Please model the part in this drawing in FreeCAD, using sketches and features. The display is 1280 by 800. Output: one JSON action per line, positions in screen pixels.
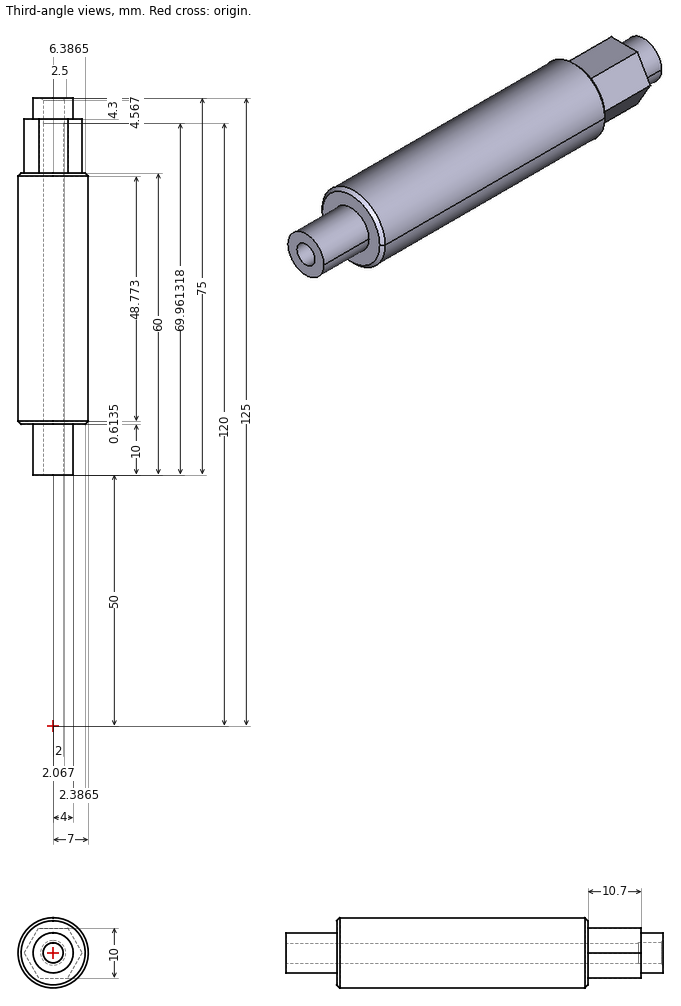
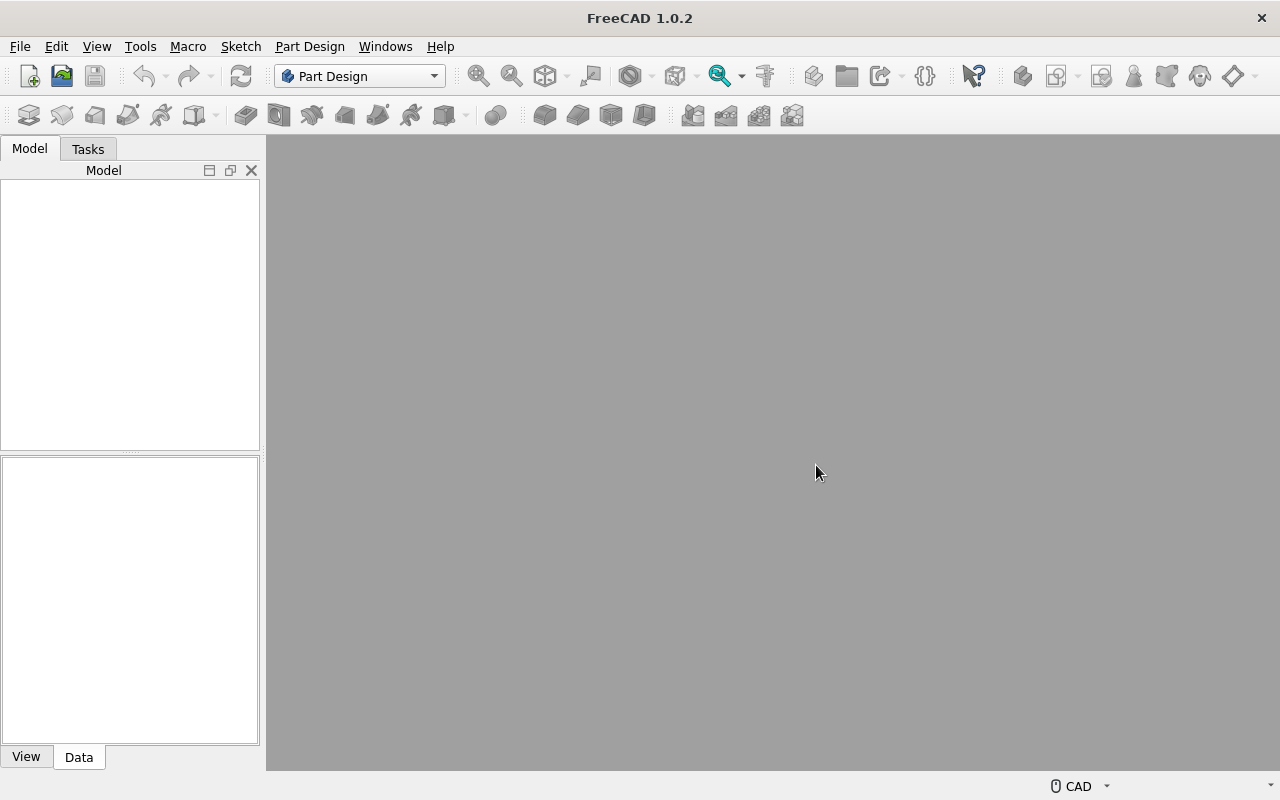
{"action": "left_click", "coordinate": [29, 76]}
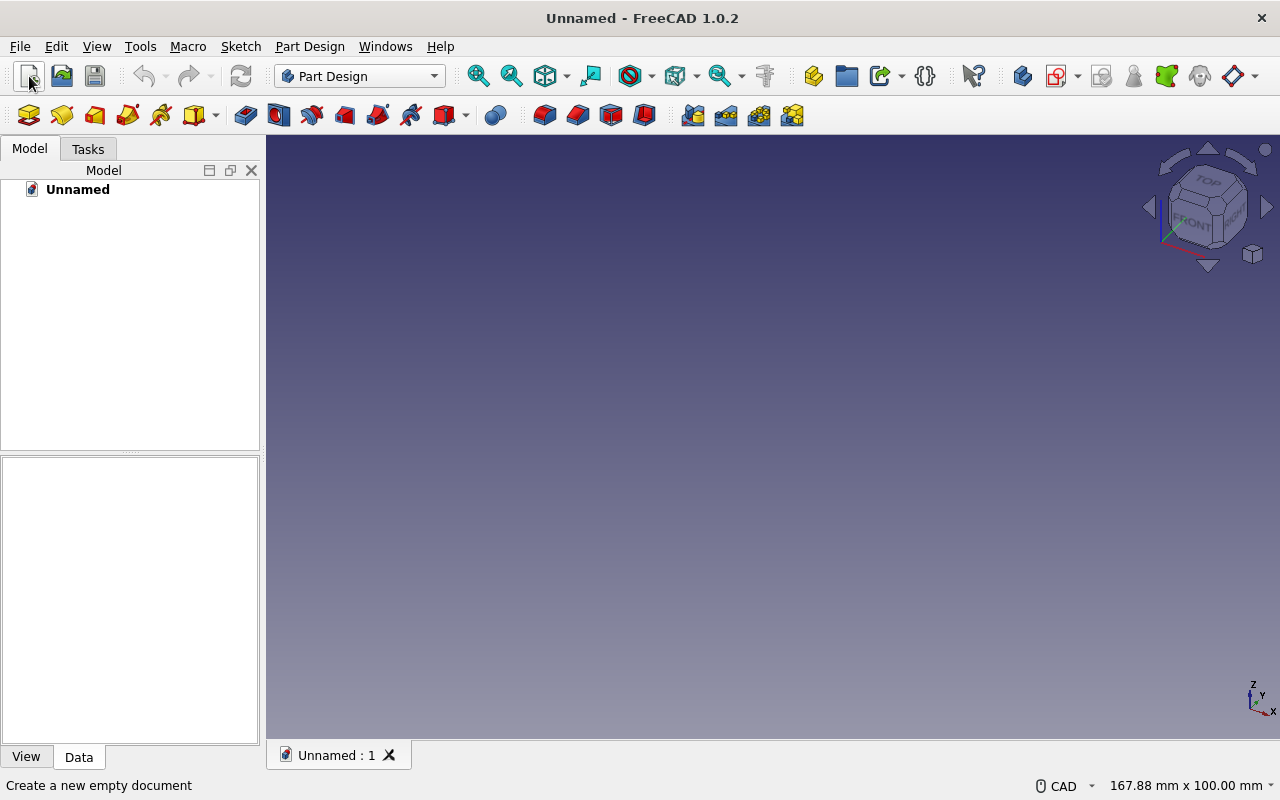
{"action": "left_click", "coordinate": [1056, 76]}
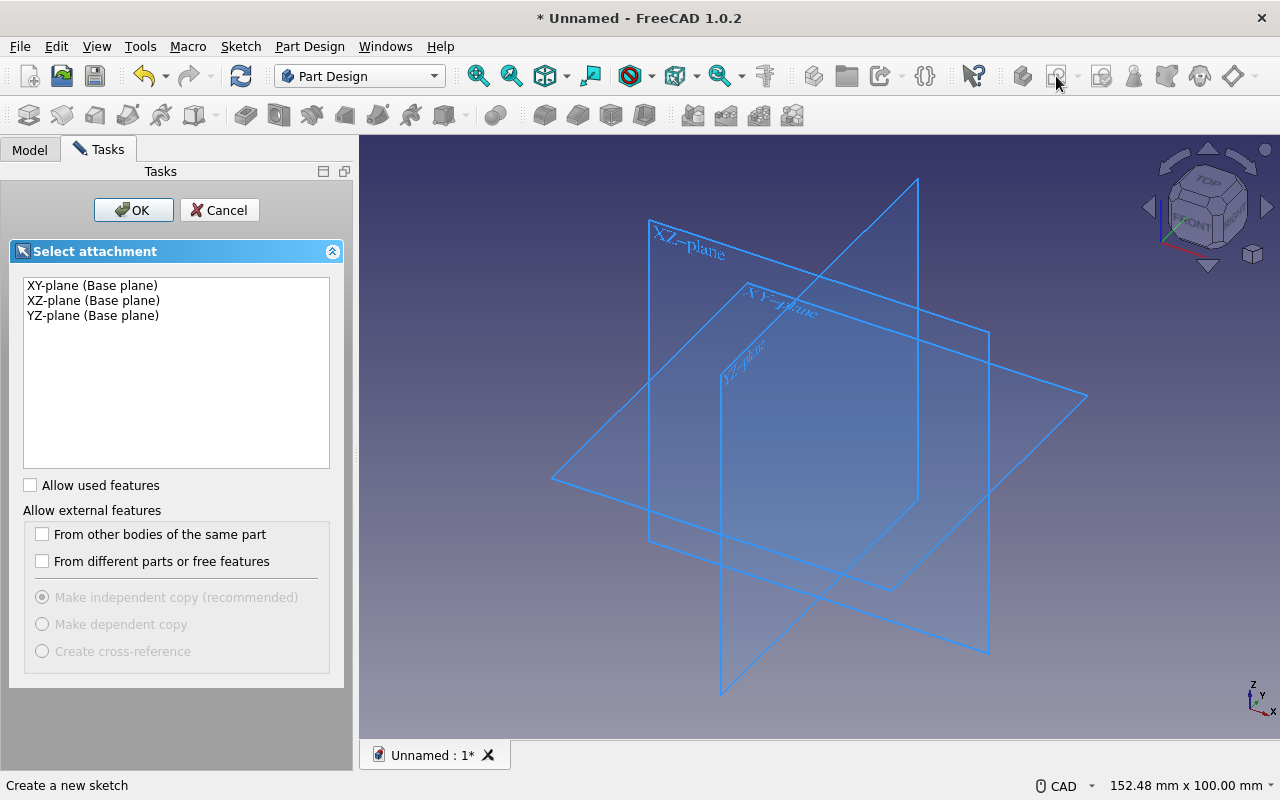
{"action": "left_click", "coordinate": [84, 286]}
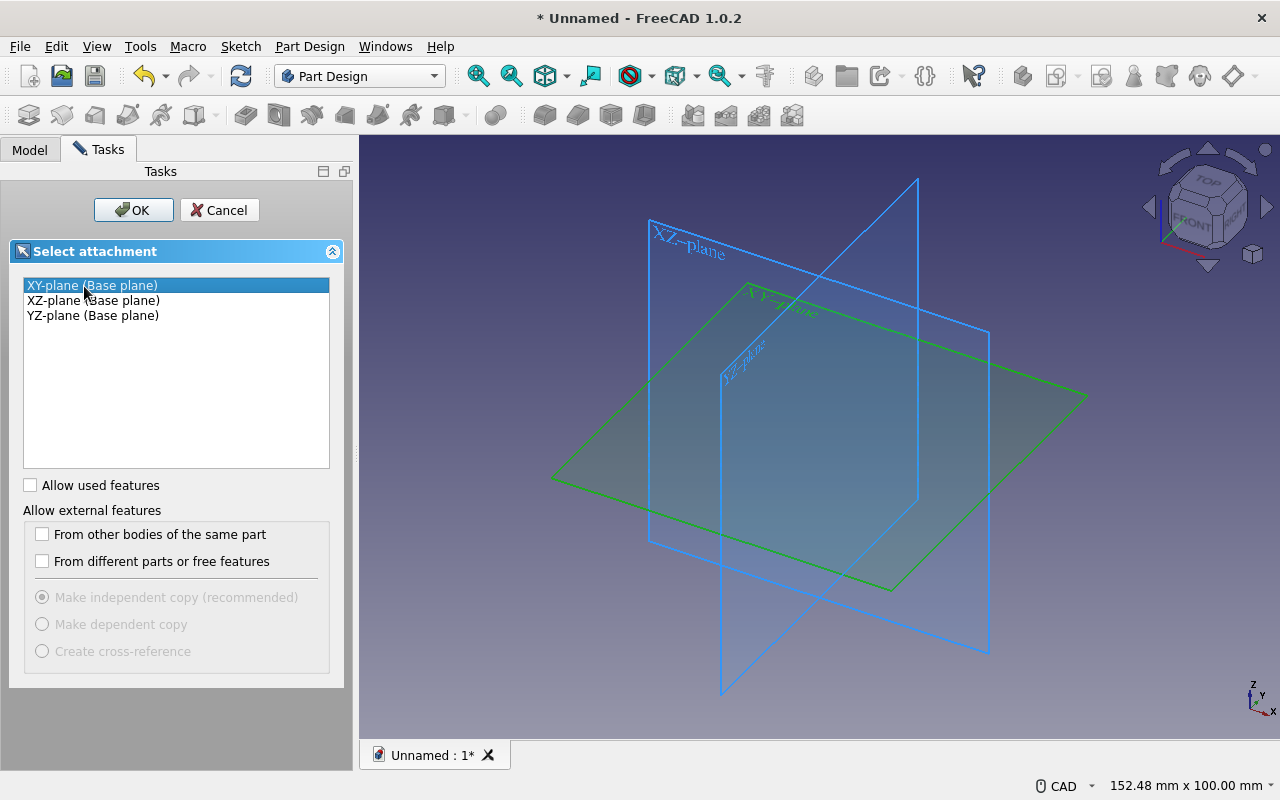
{"action": "left_click", "coordinate": [134, 210]}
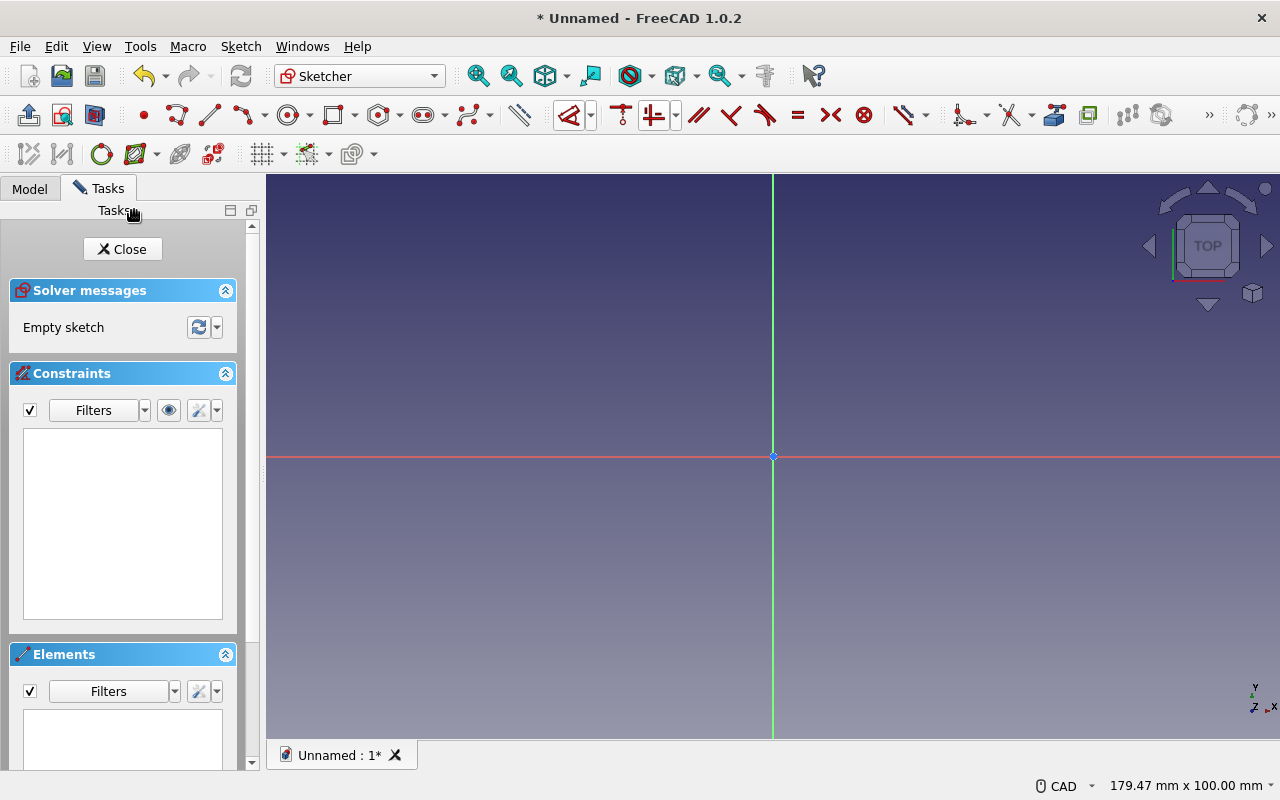
{"action": "scroll", "coordinate": [597, 711], "scroll_direction": "down", "scroll_amount": 3}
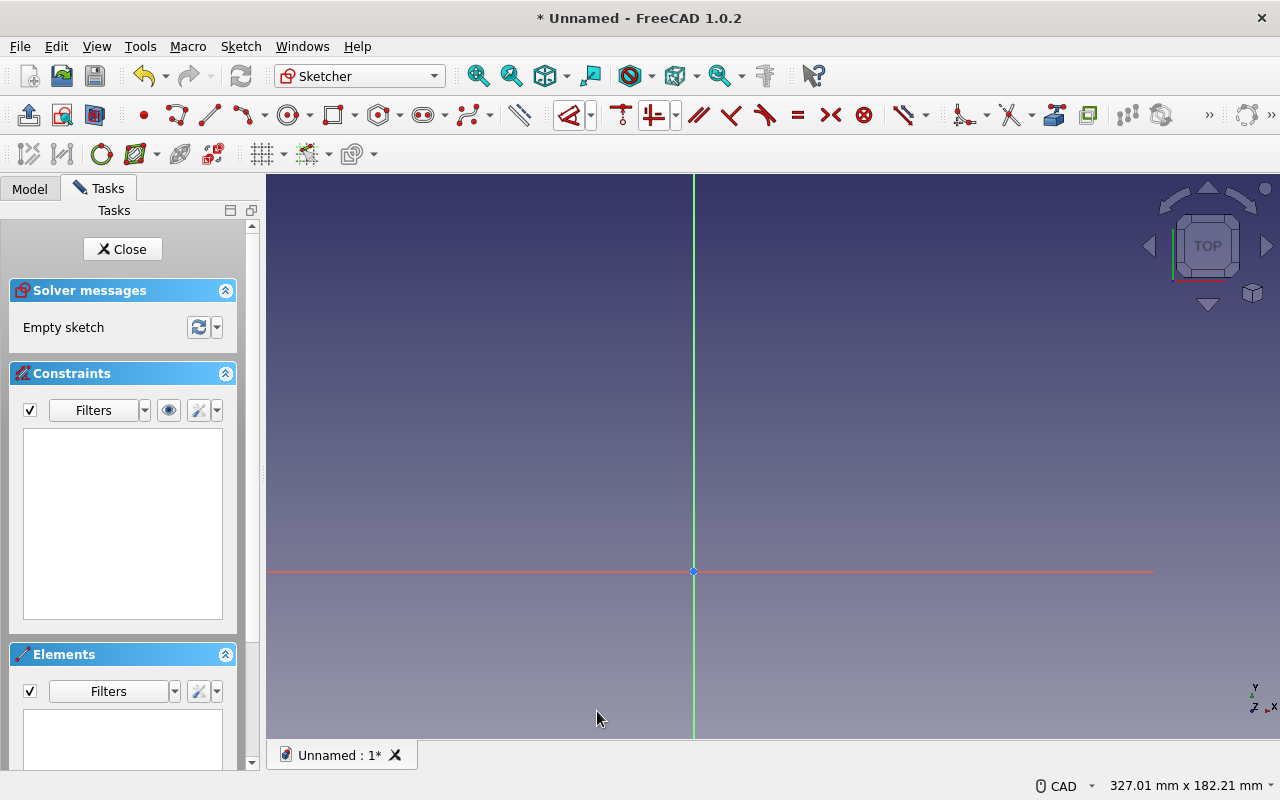
{"action": "left_click", "coordinate": [177, 116]}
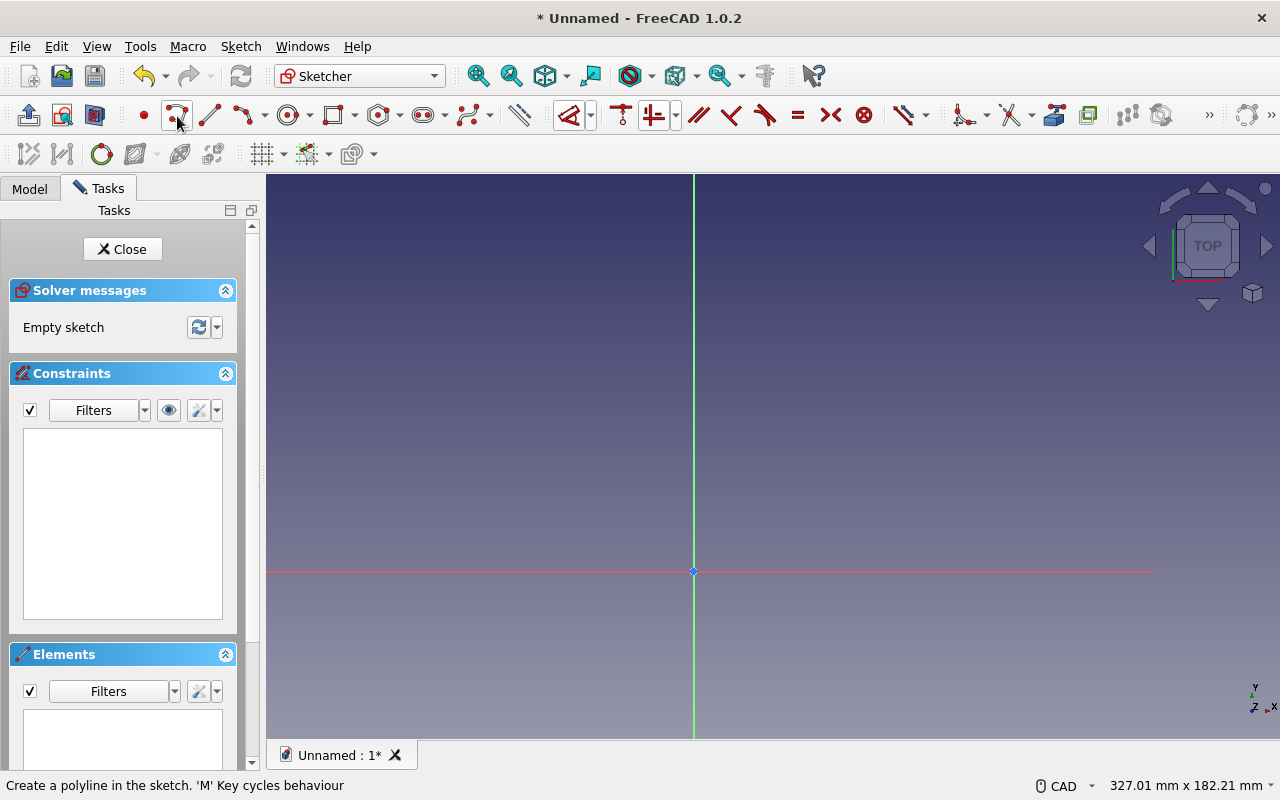
{"action": "left_click", "coordinate": [694, 417]}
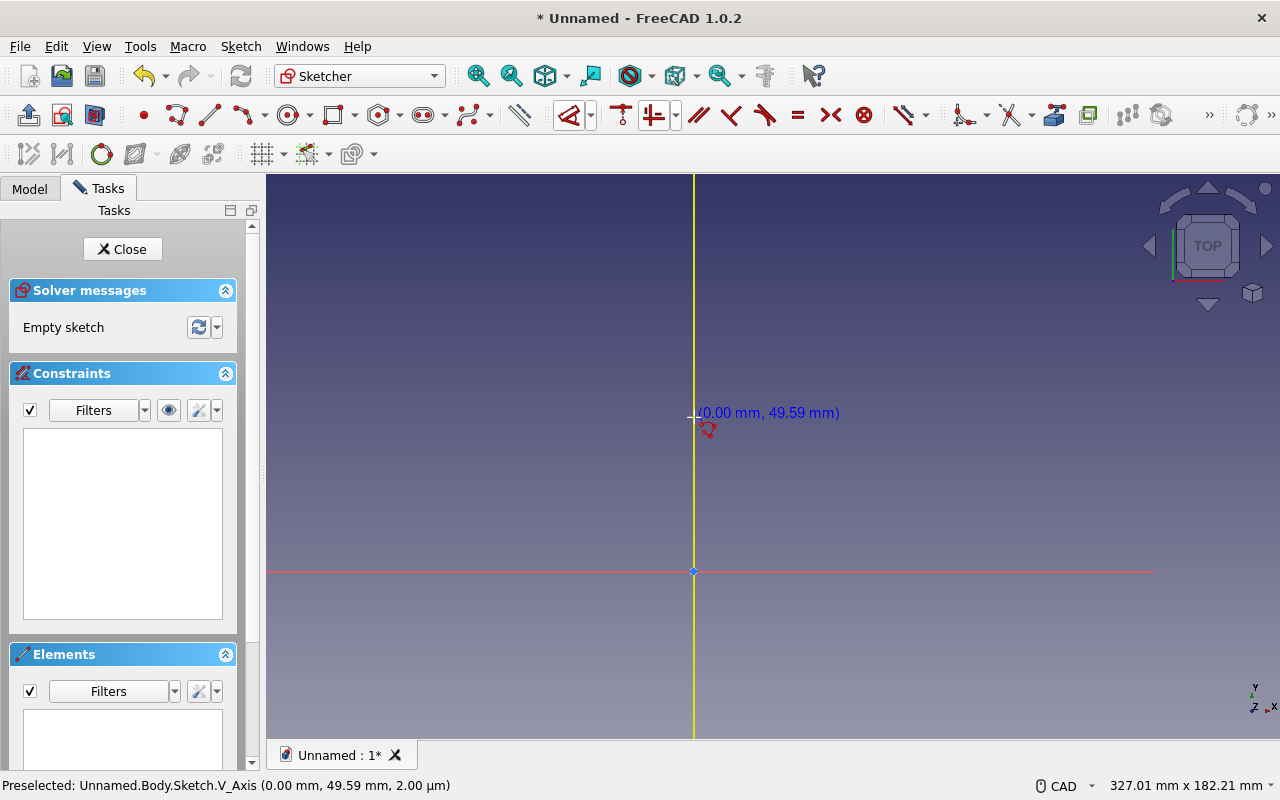
{"action": "scroll", "coordinate": [706, 417], "scroll_direction": "up", "scroll_amount": 2}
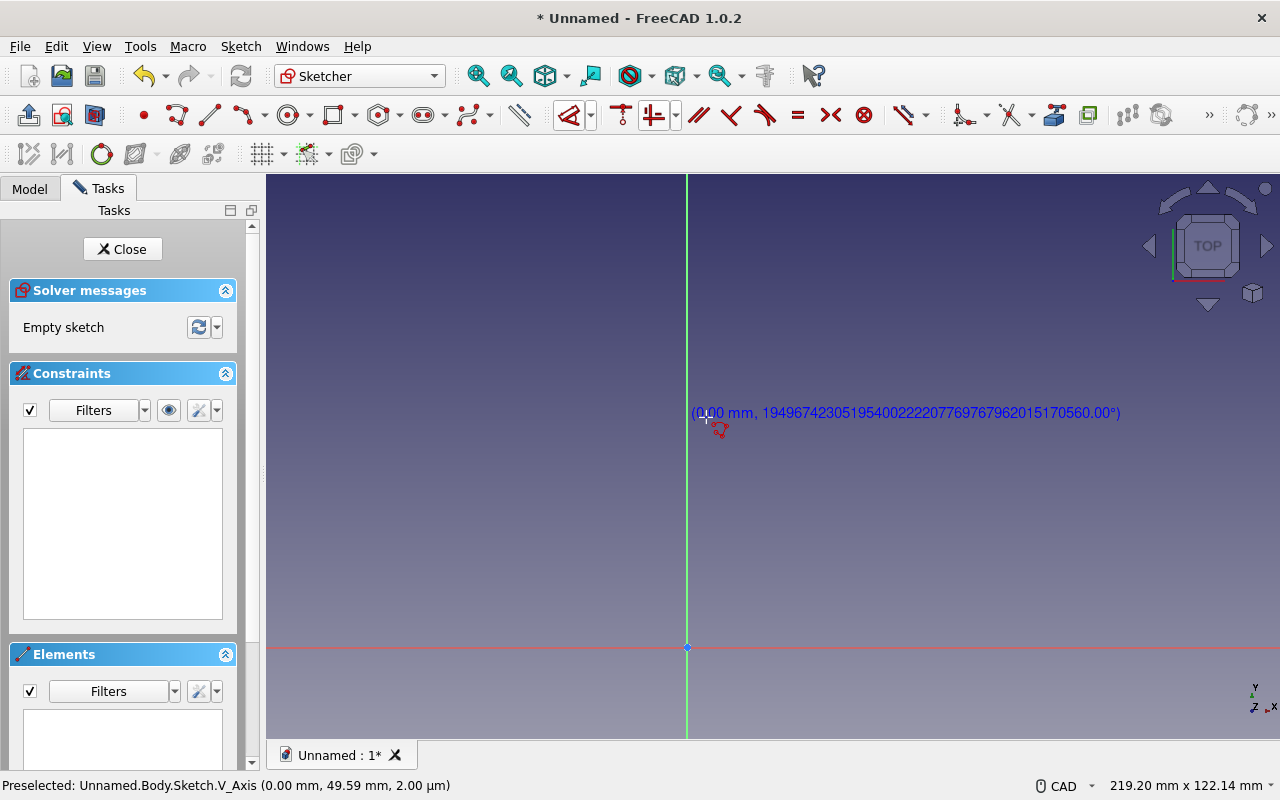
{"action": "left_click", "coordinate": [706, 417]}
{"action": "left_click", "coordinate": [706, 370]}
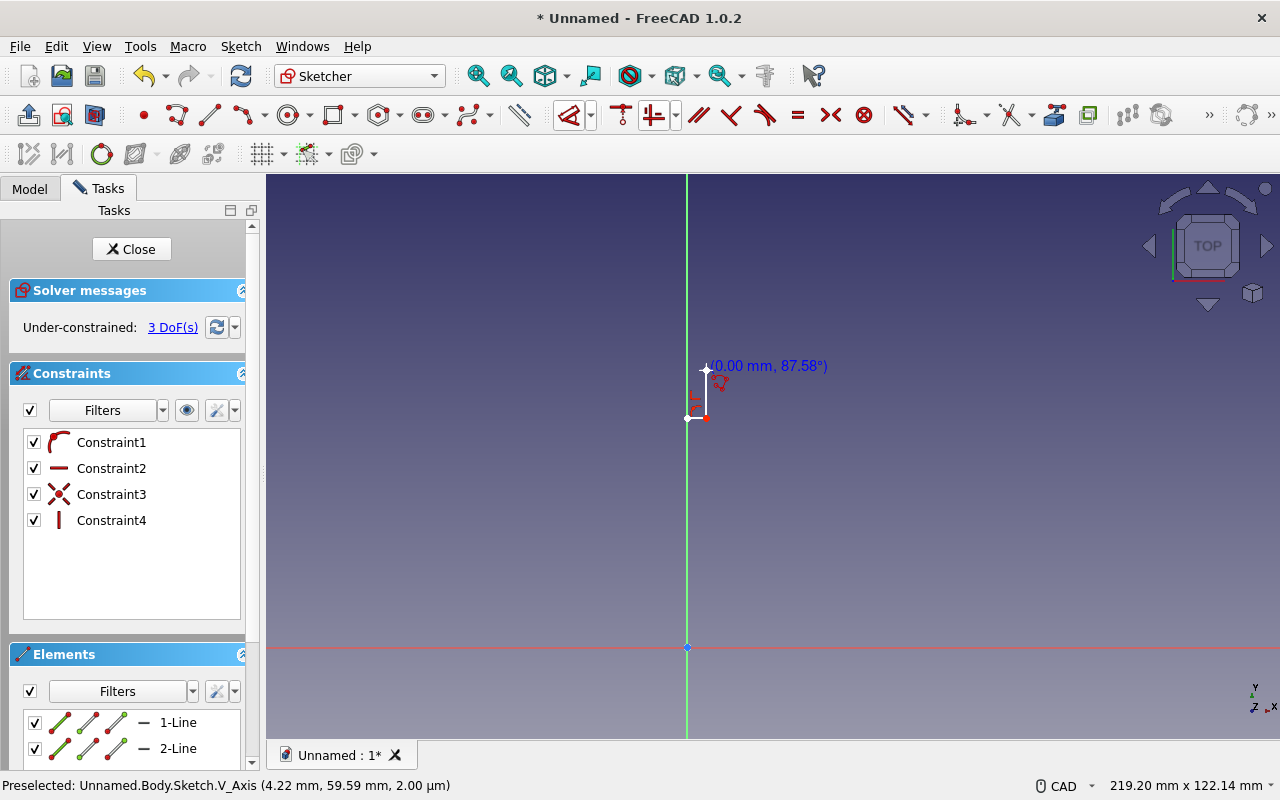
{"action": "scroll", "coordinate": [717, 370], "scroll_direction": "up", "scroll_amount": 2}